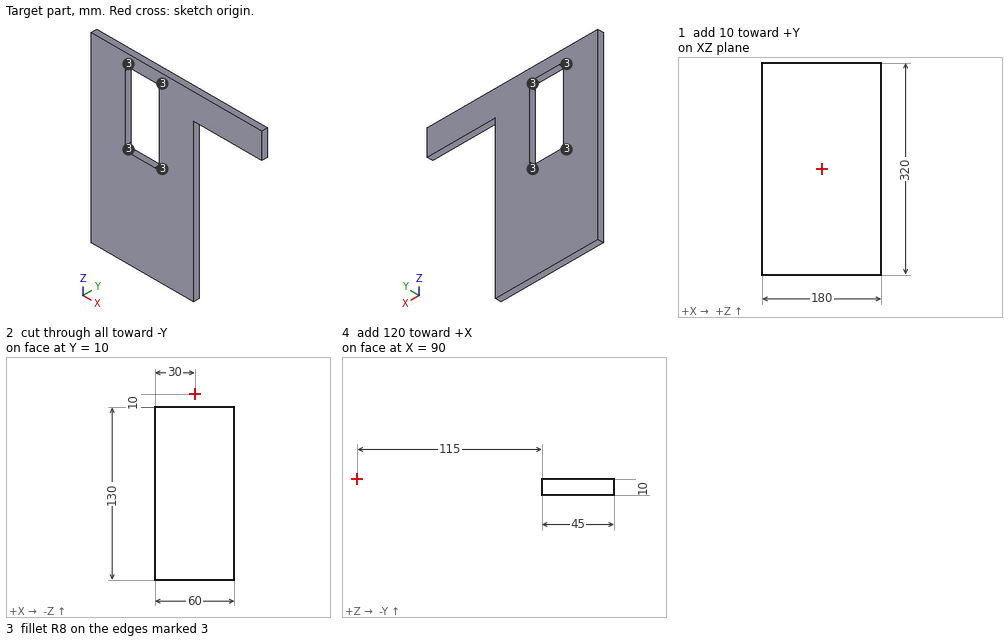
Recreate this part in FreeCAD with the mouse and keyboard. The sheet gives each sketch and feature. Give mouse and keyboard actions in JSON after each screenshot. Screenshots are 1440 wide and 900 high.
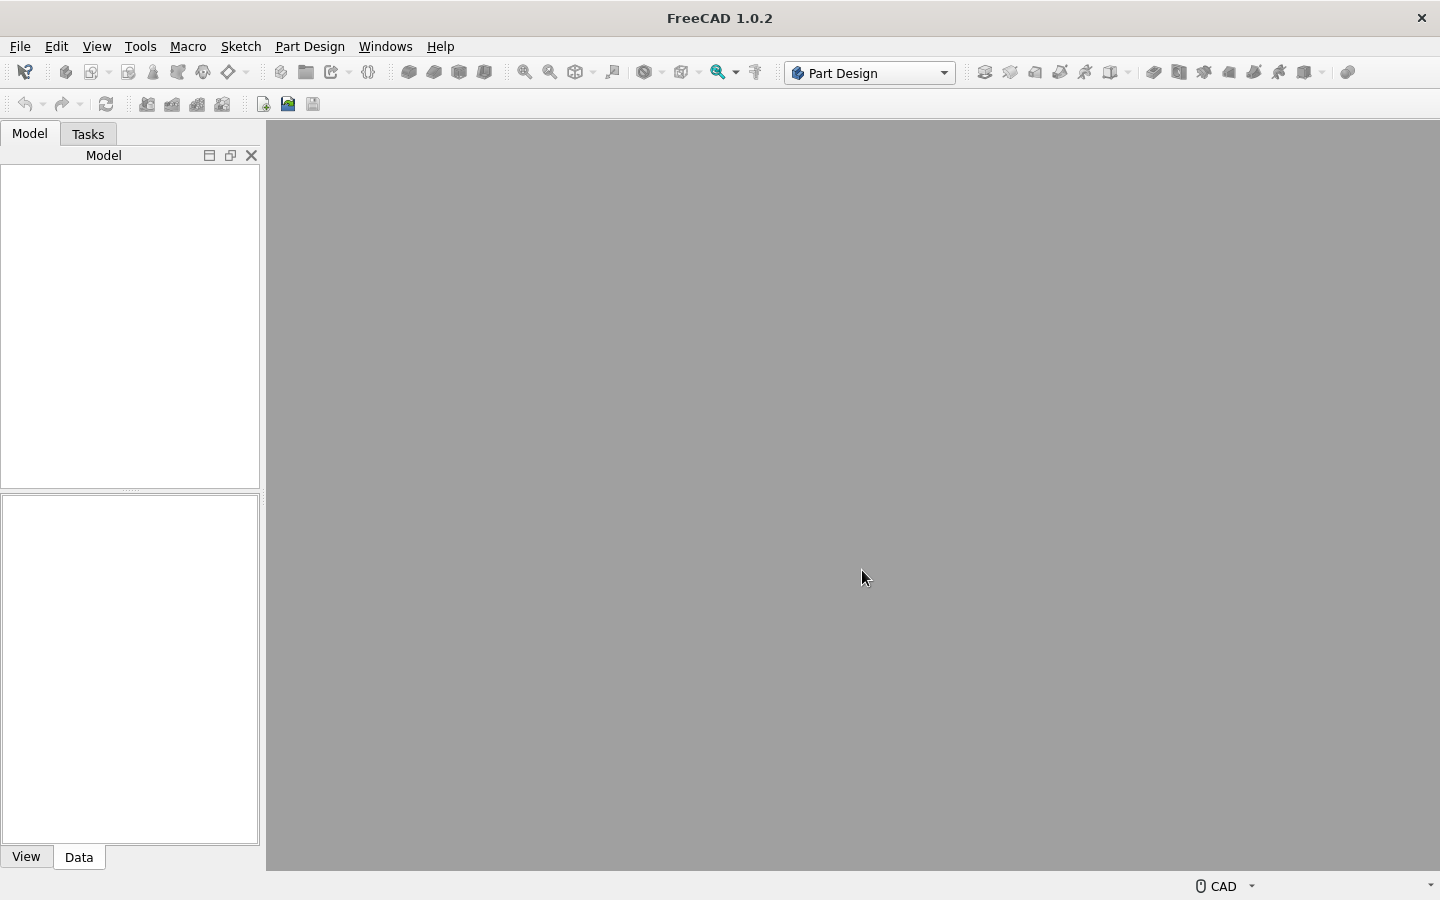
{"action": "left_click", "coordinate": [263, 104]}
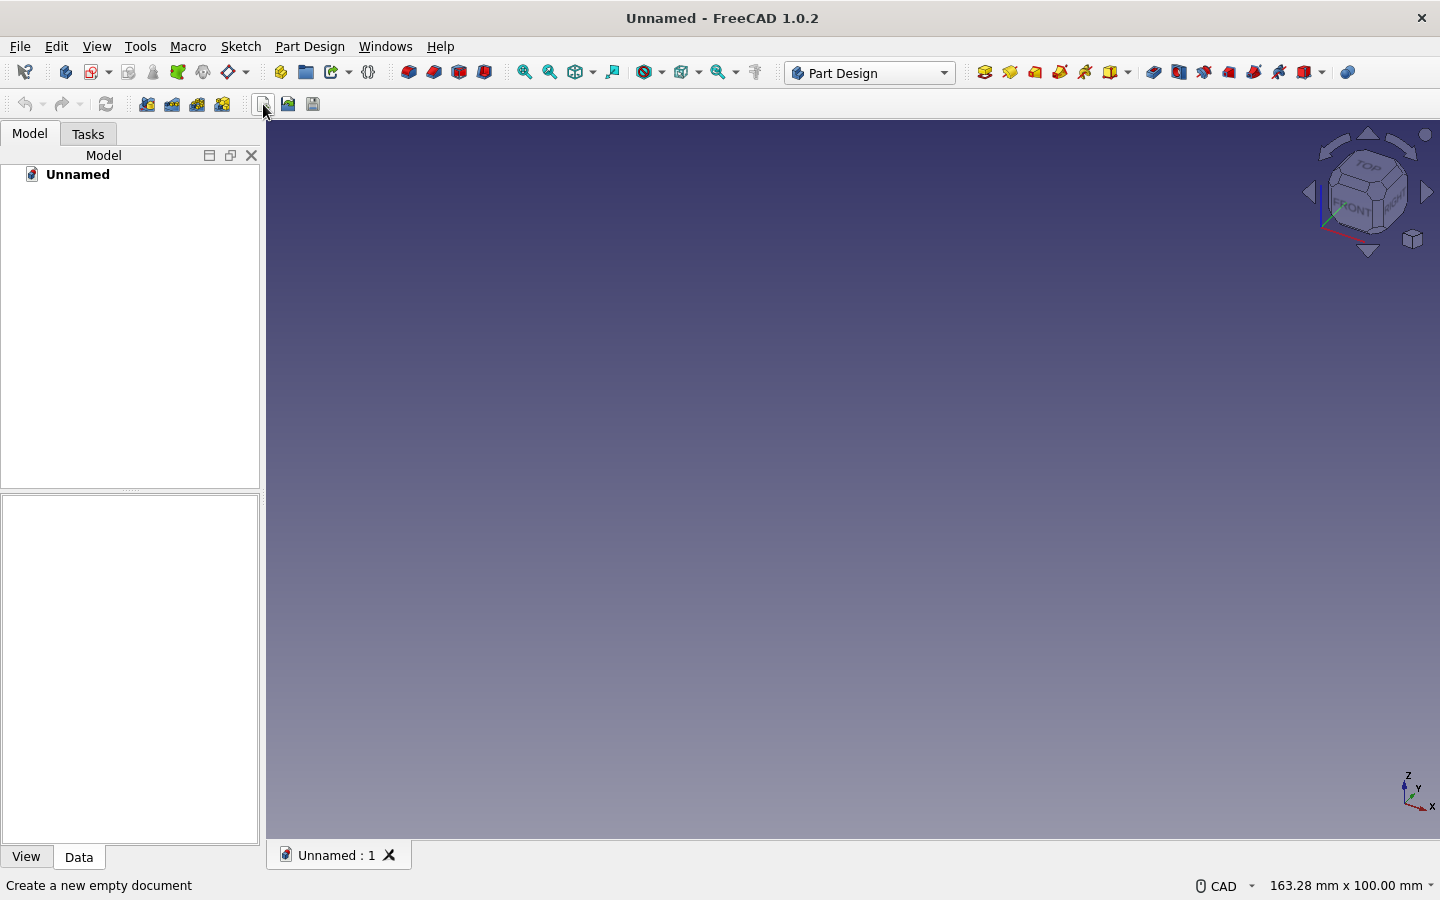
{"action": "left_click", "coordinate": [90, 72]}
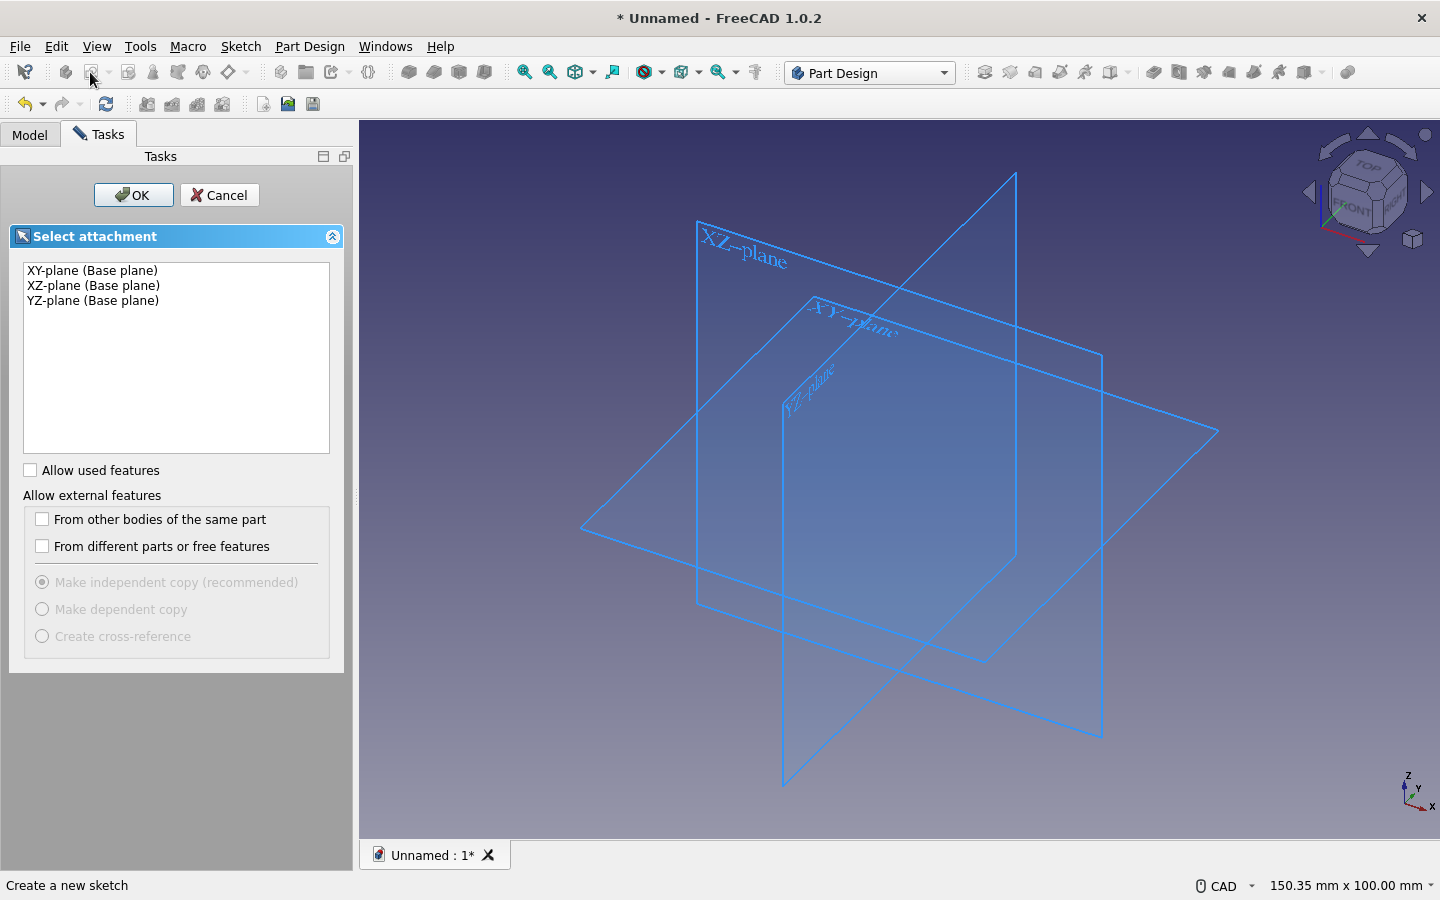
{"action": "left_click", "coordinate": [84, 286]}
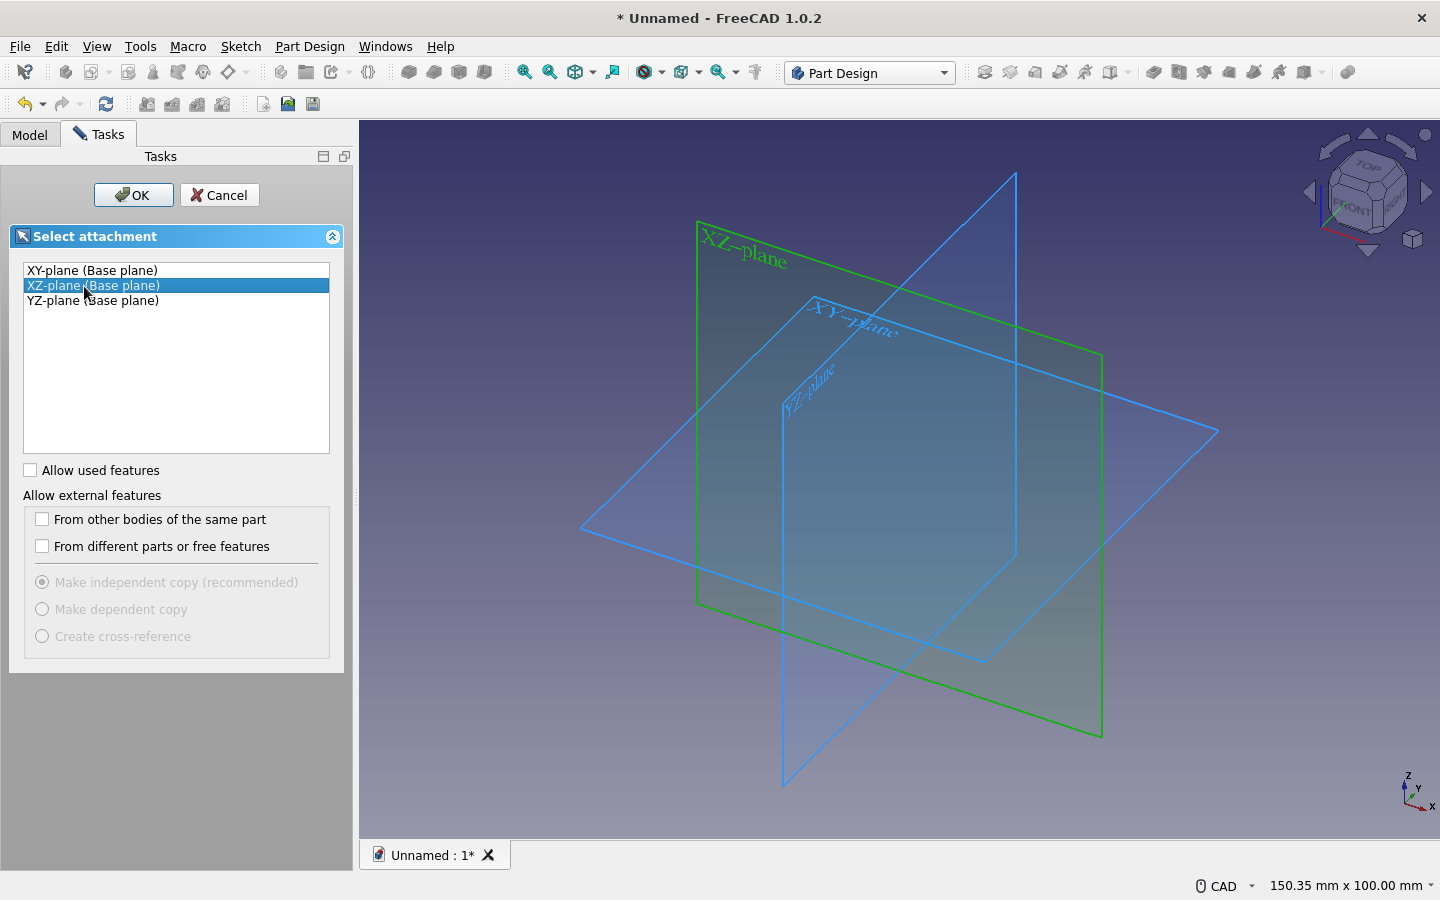
{"action": "left_click", "coordinate": [134, 195]}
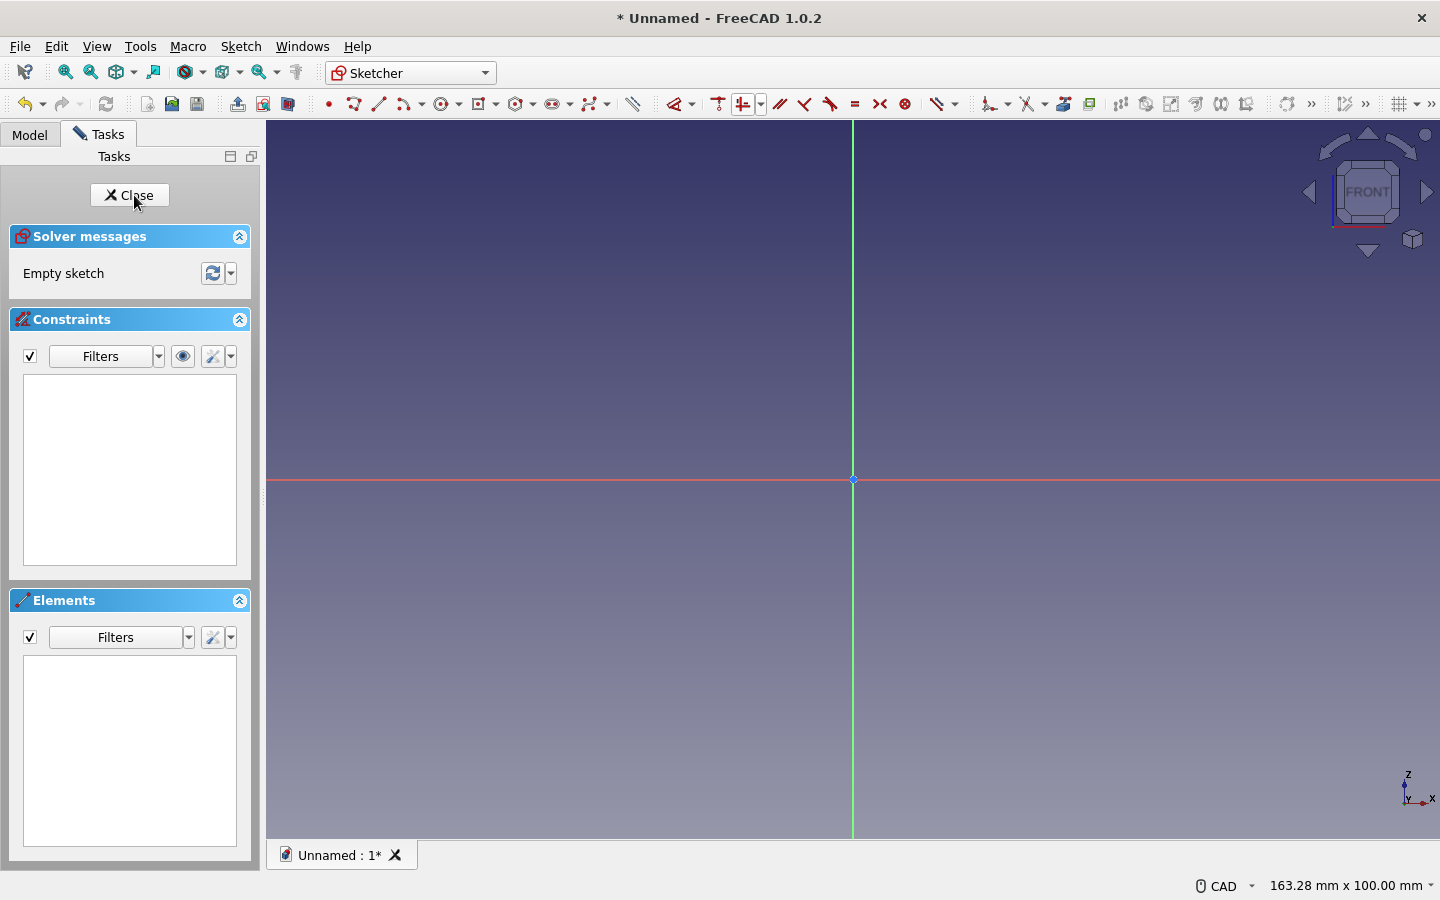
{"action": "scroll", "coordinate": [767, 480], "scroll_direction": "down", "scroll_amount": 8}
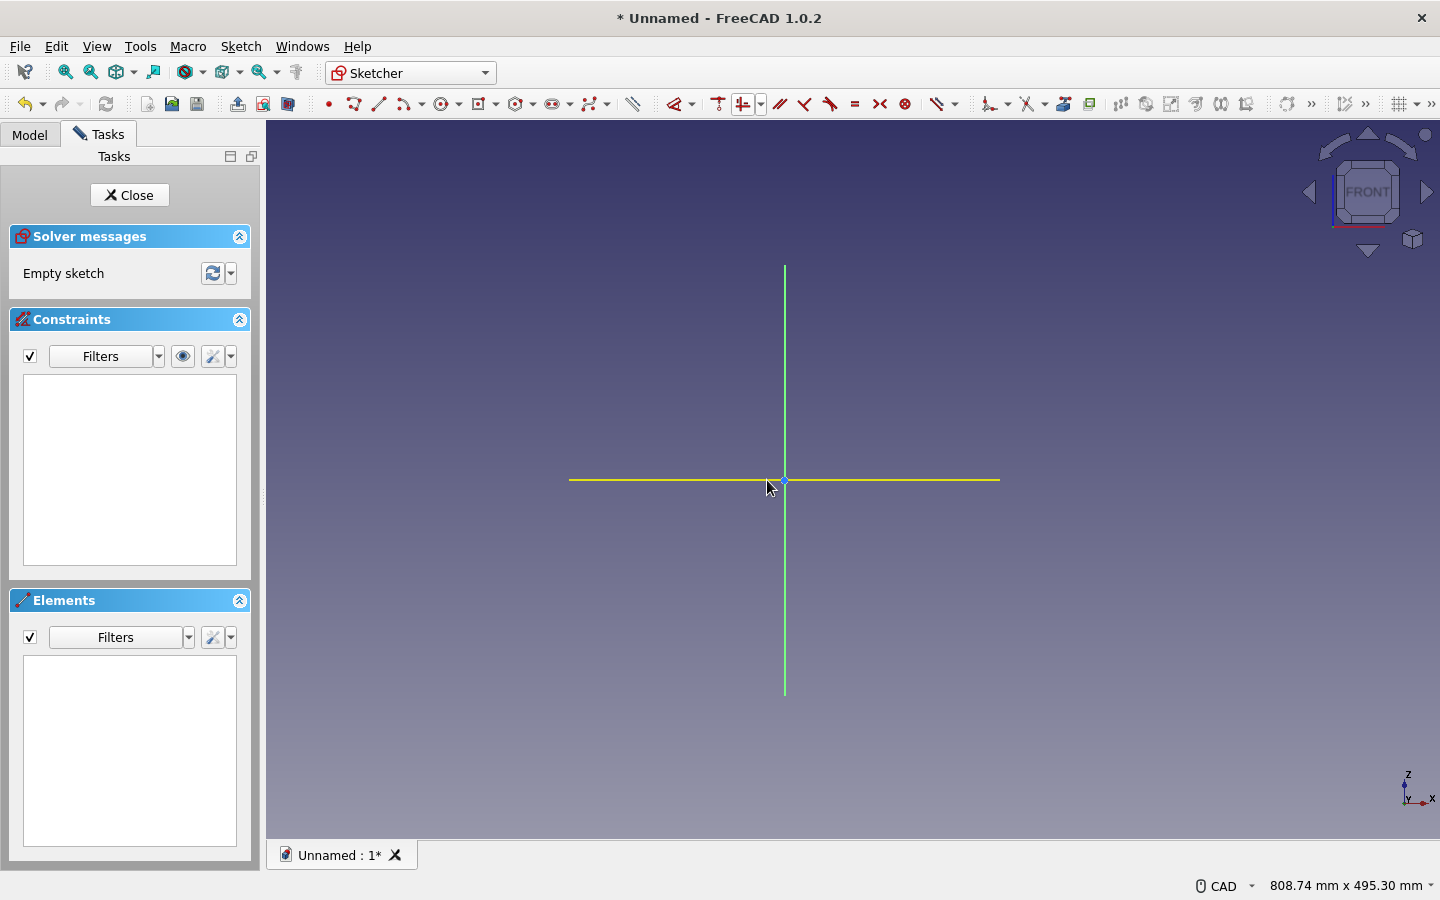
{"action": "key", "text": "g v"}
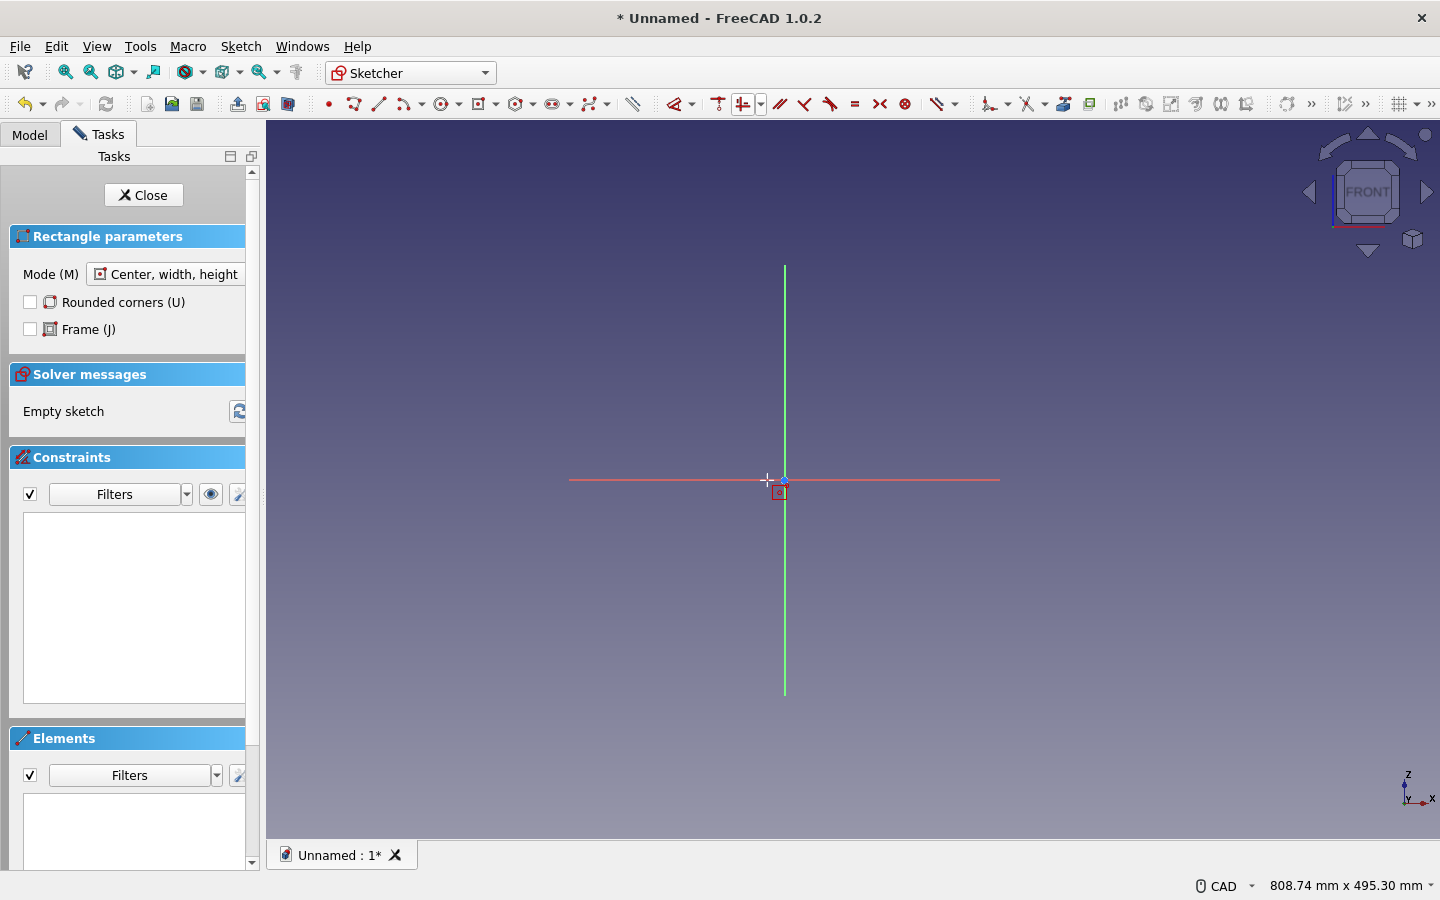
{"action": "left_click", "coordinate": [785, 480]}
{"action": "left_click", "coordinate": [915, 248]}
{"action": "key", "text": "Escape"}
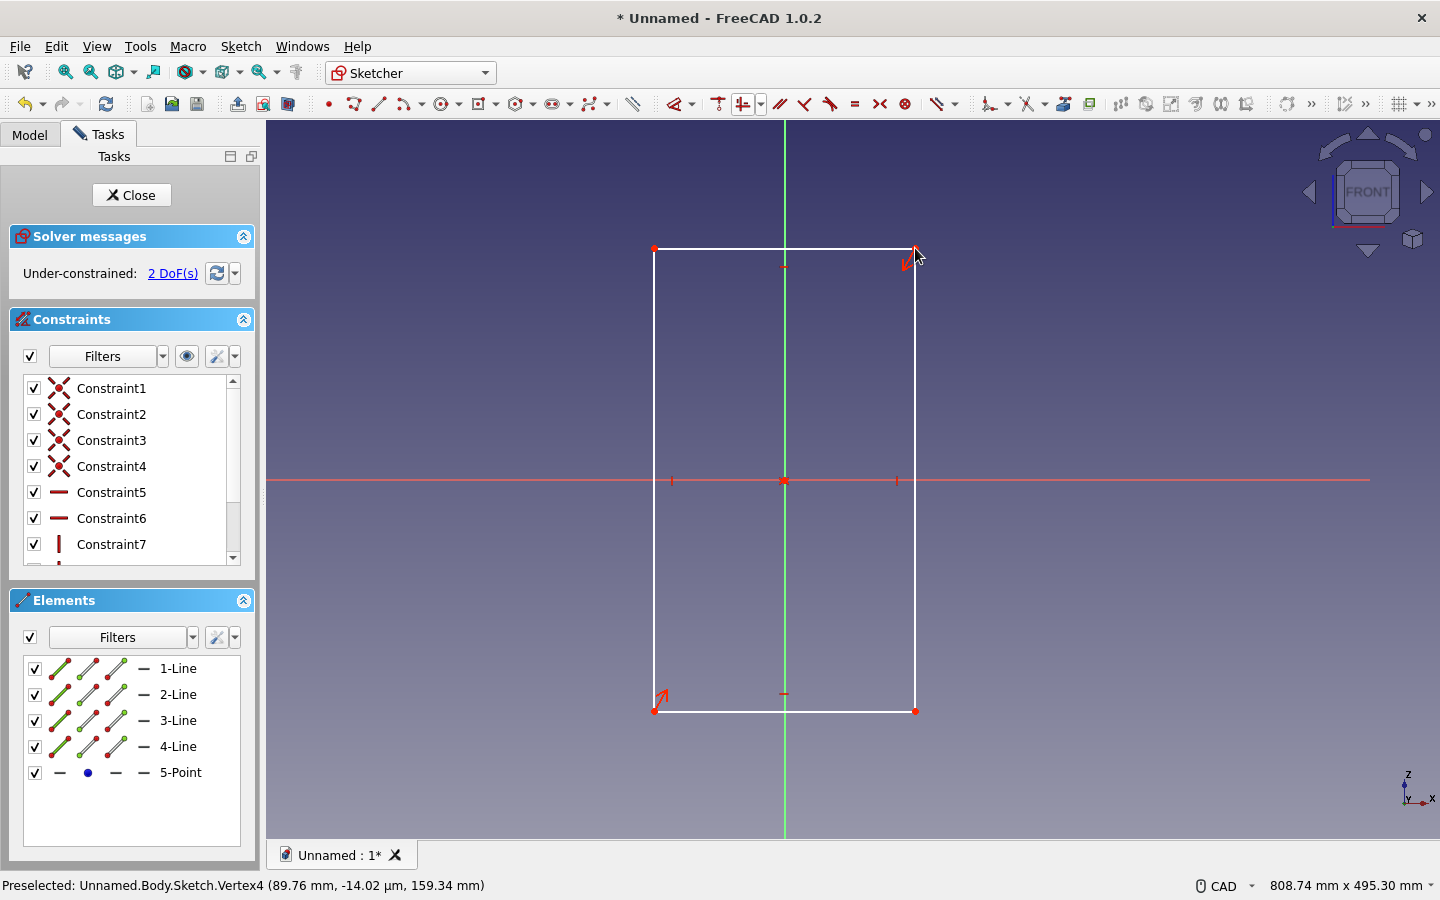
{"action": "key", "text": "d"}